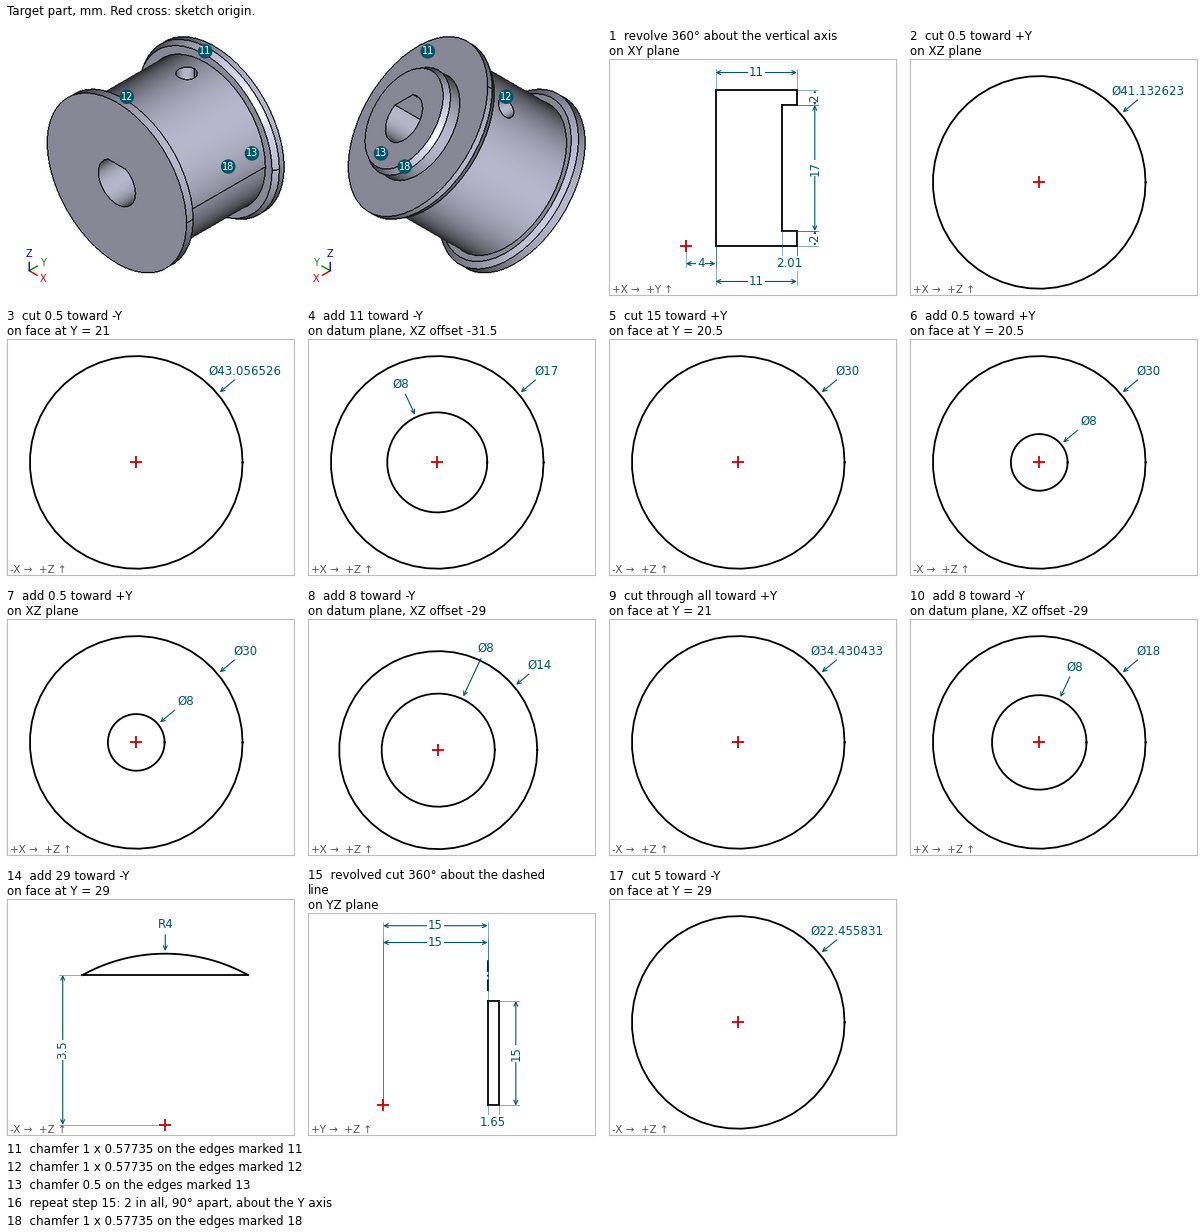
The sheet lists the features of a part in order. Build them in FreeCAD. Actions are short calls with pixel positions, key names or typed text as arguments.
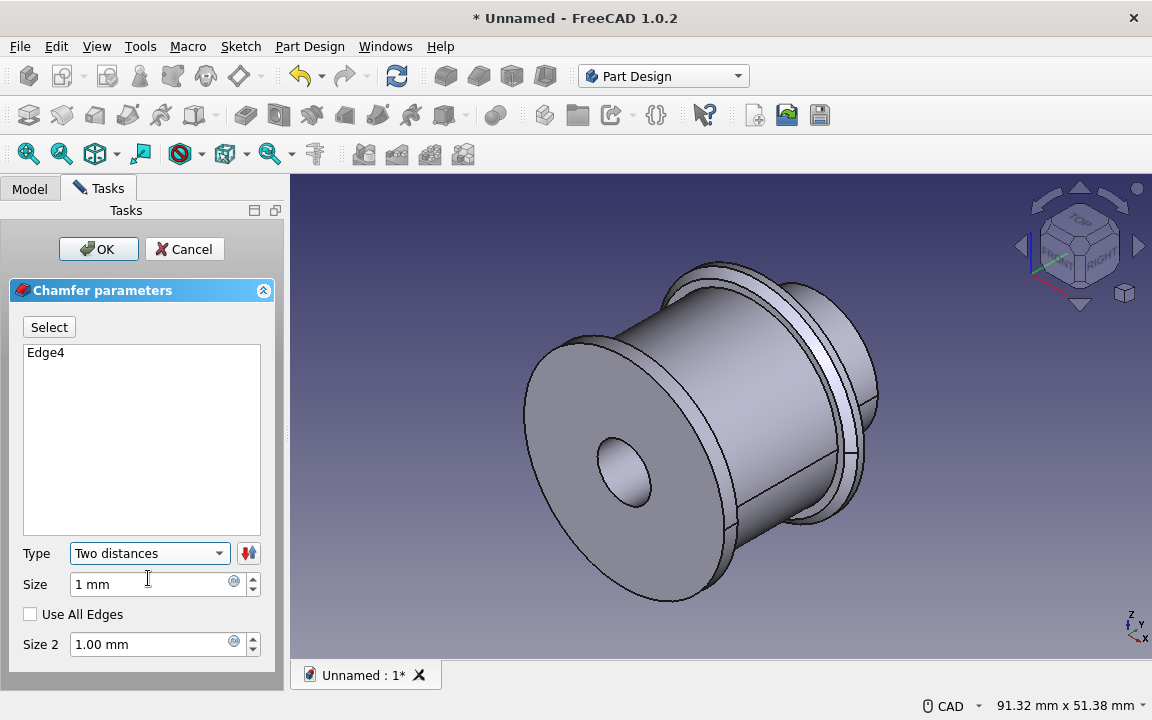
triple_click(158, 644)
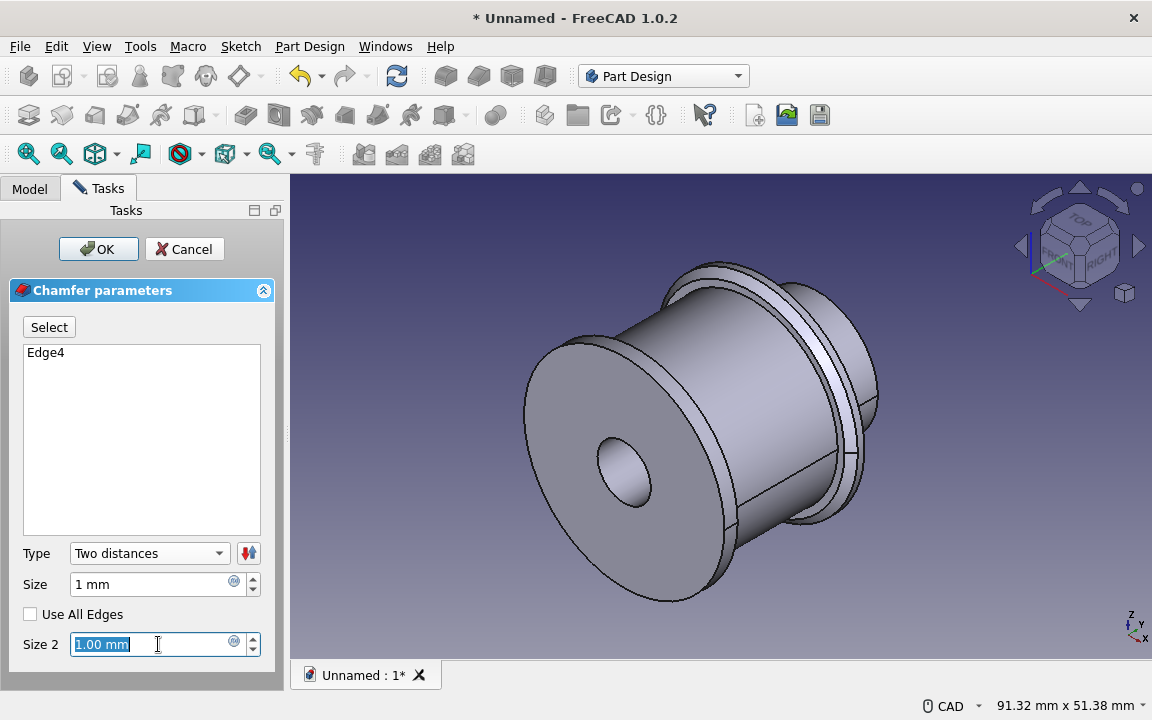
text(0.57735)
key(Tab)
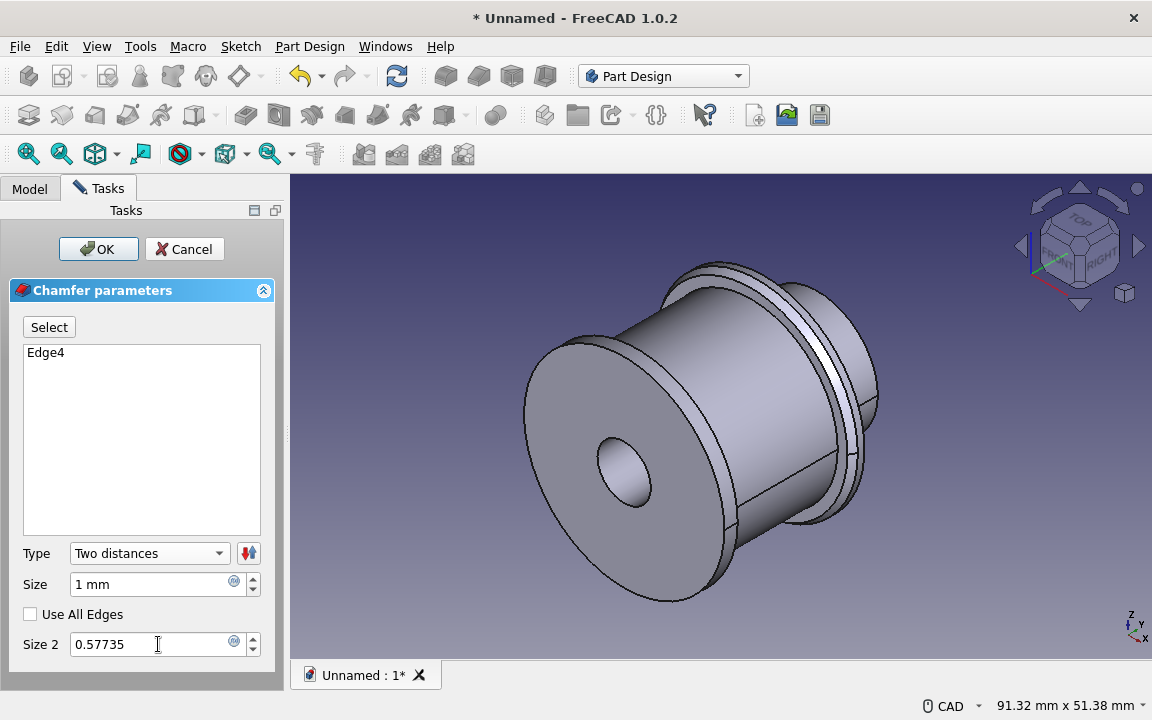
click(99, 249)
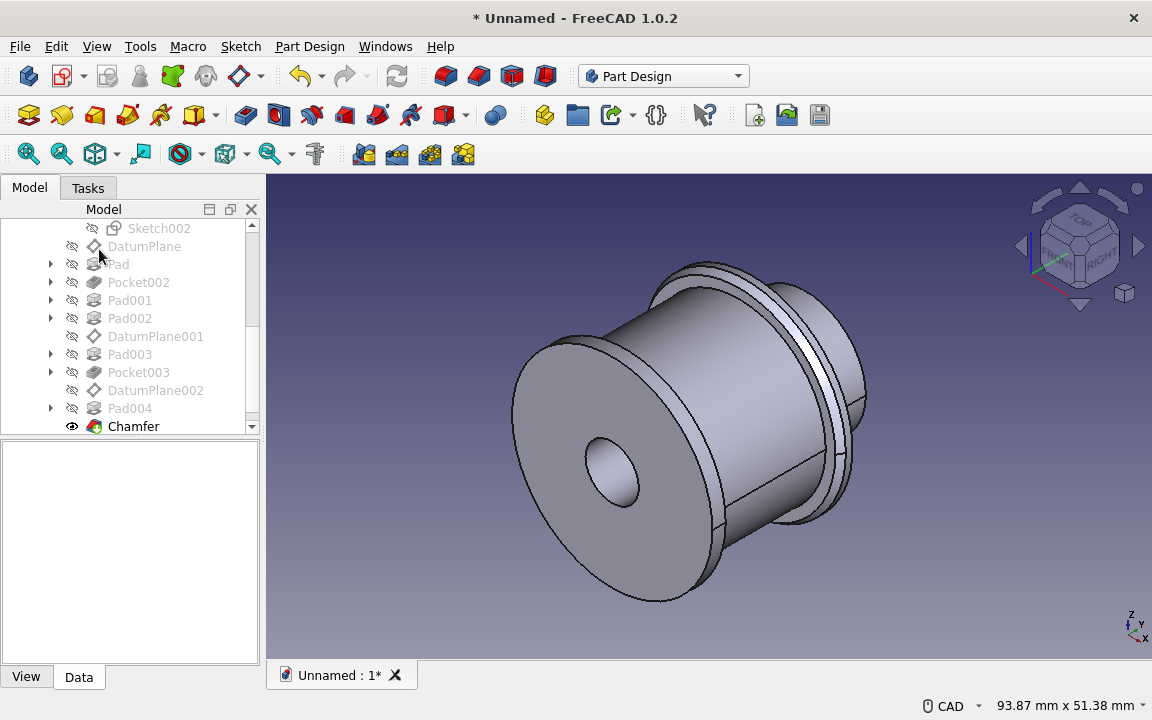
key(2)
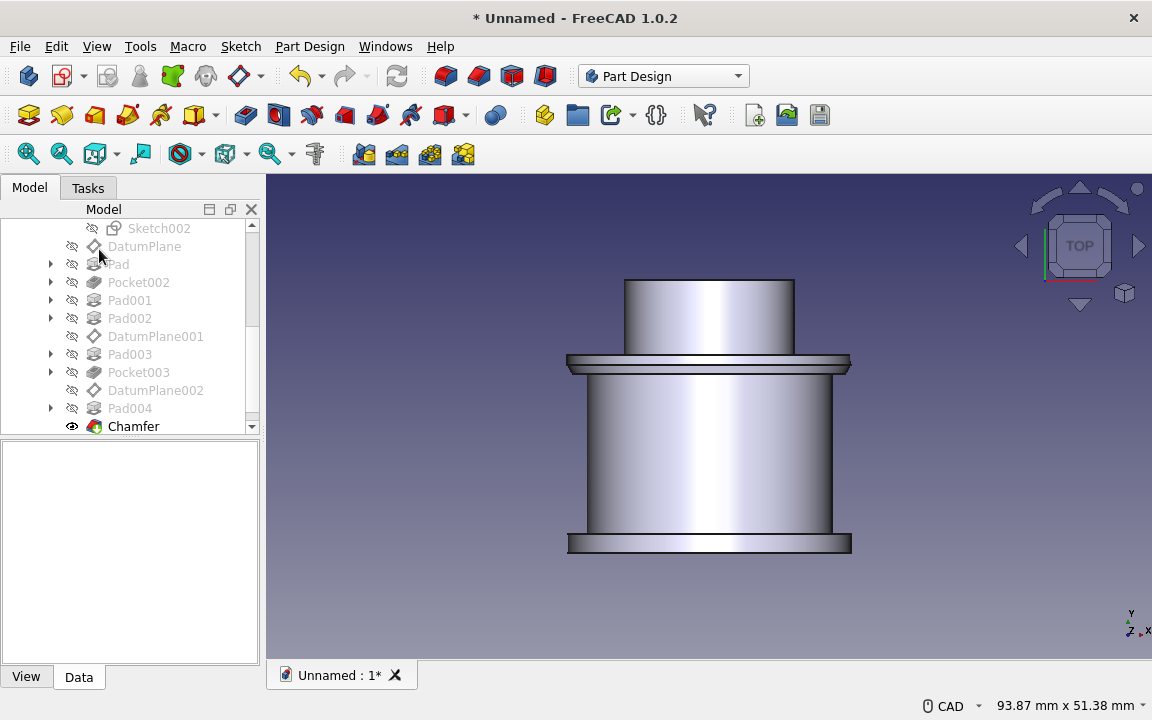
click(594, 533)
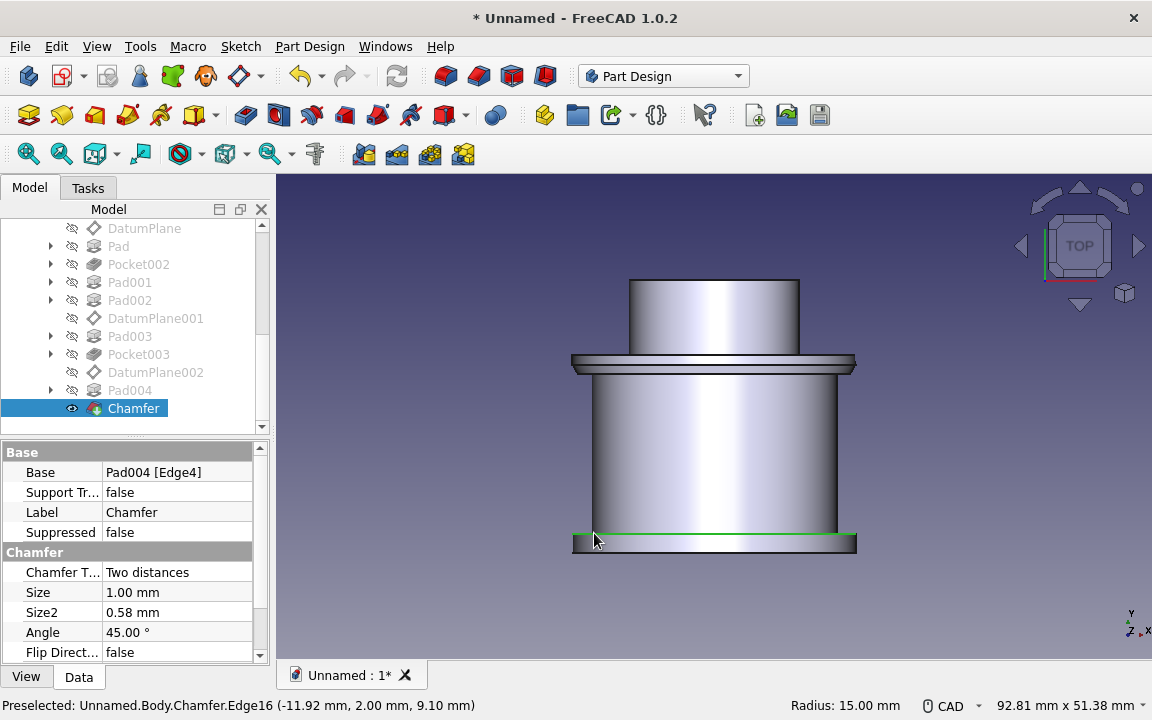
click(479, 76)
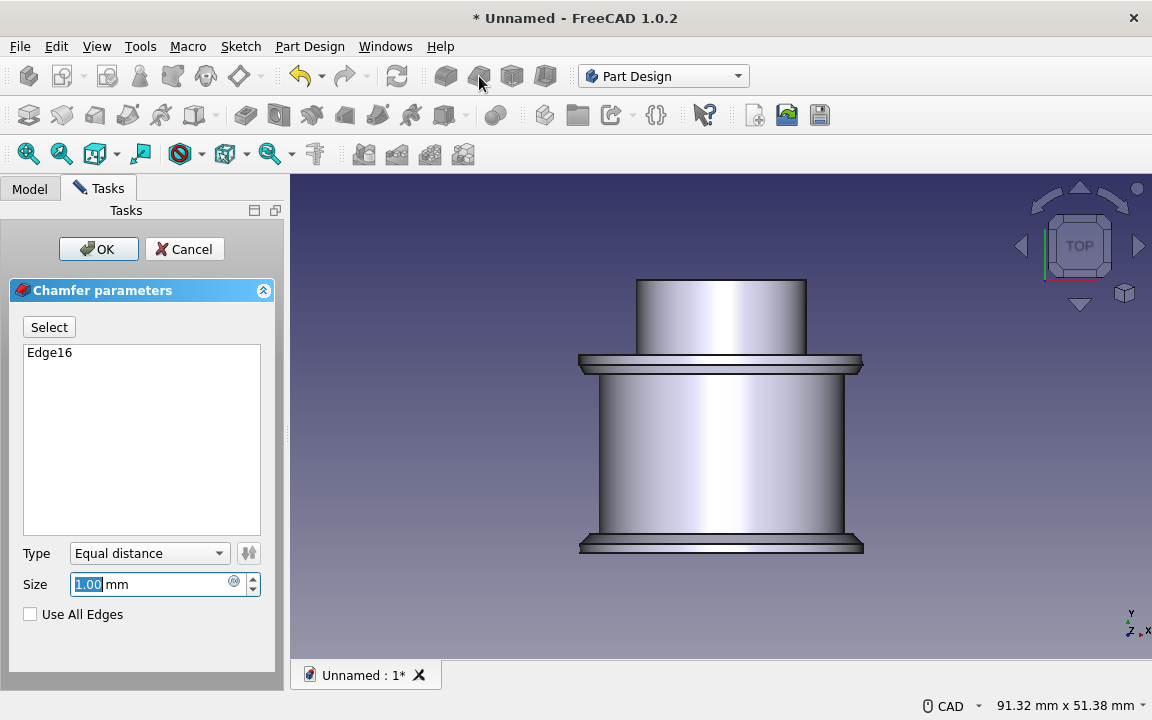
text(1)
key(Tab)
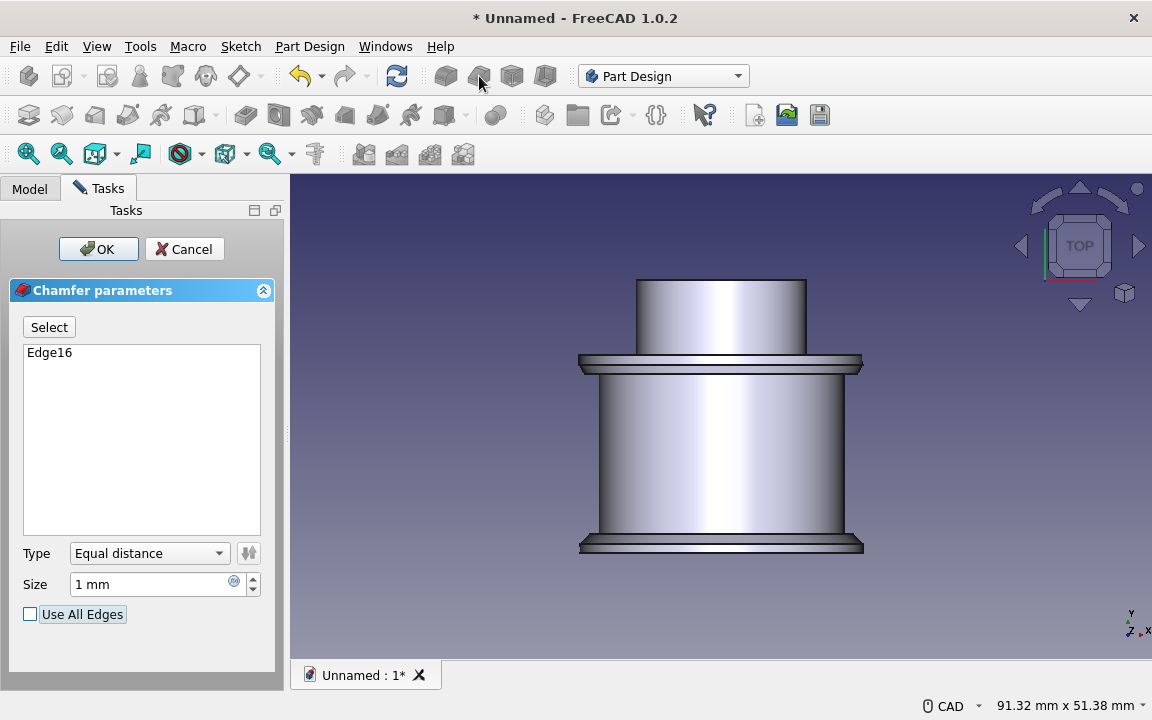
click(150, 554)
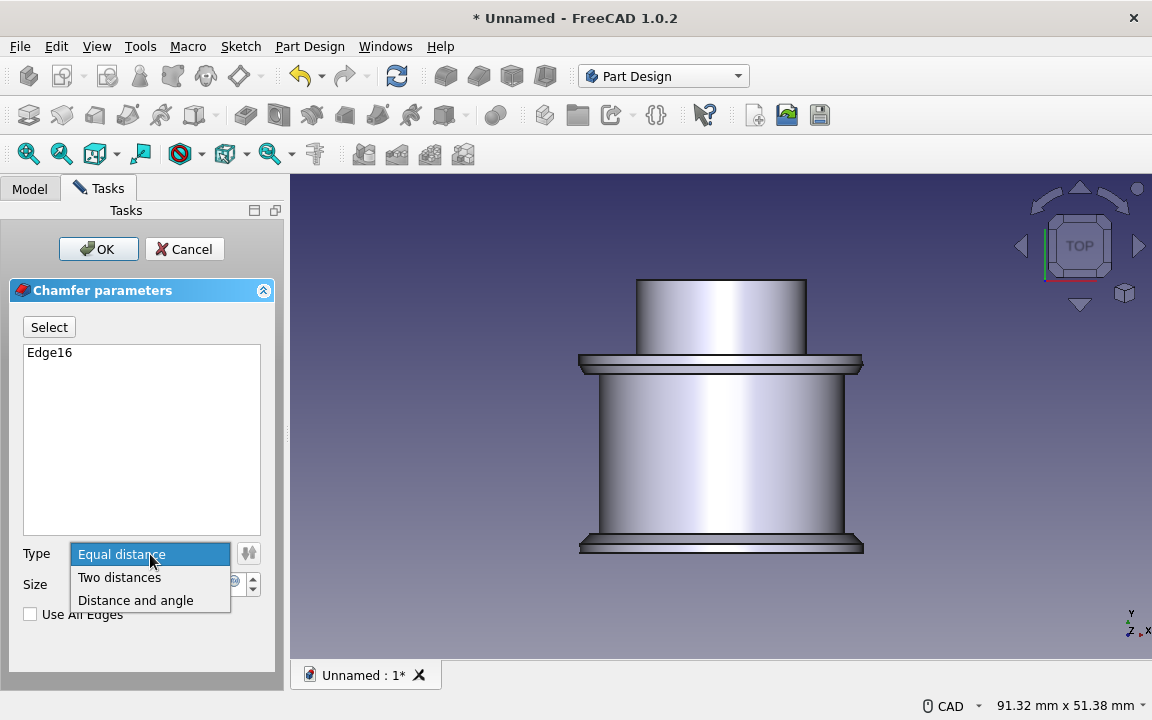
click(148, 578)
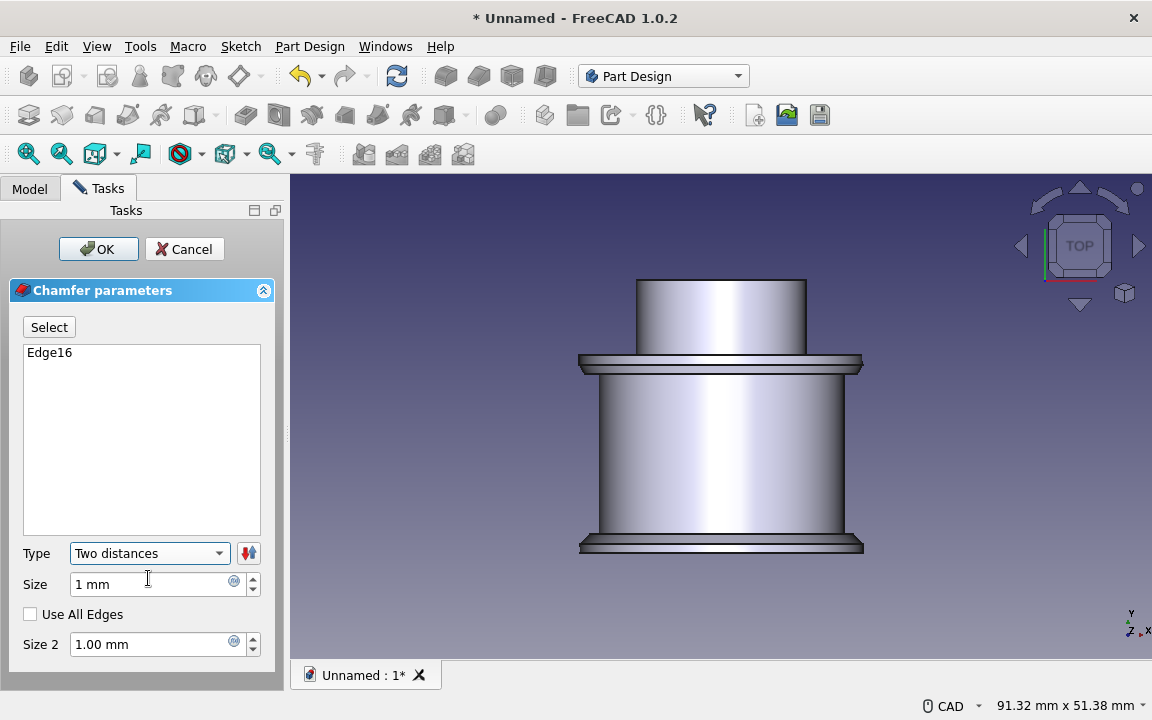
triple_click(158, 644)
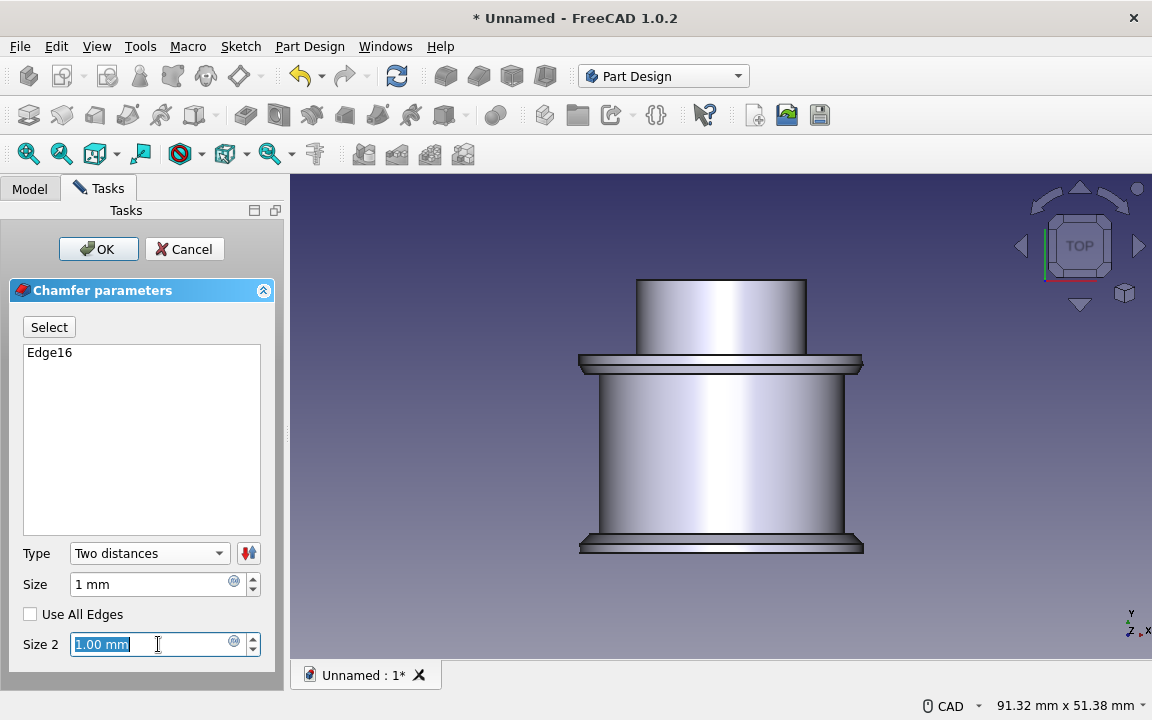
text(0.57735)
key(Tab)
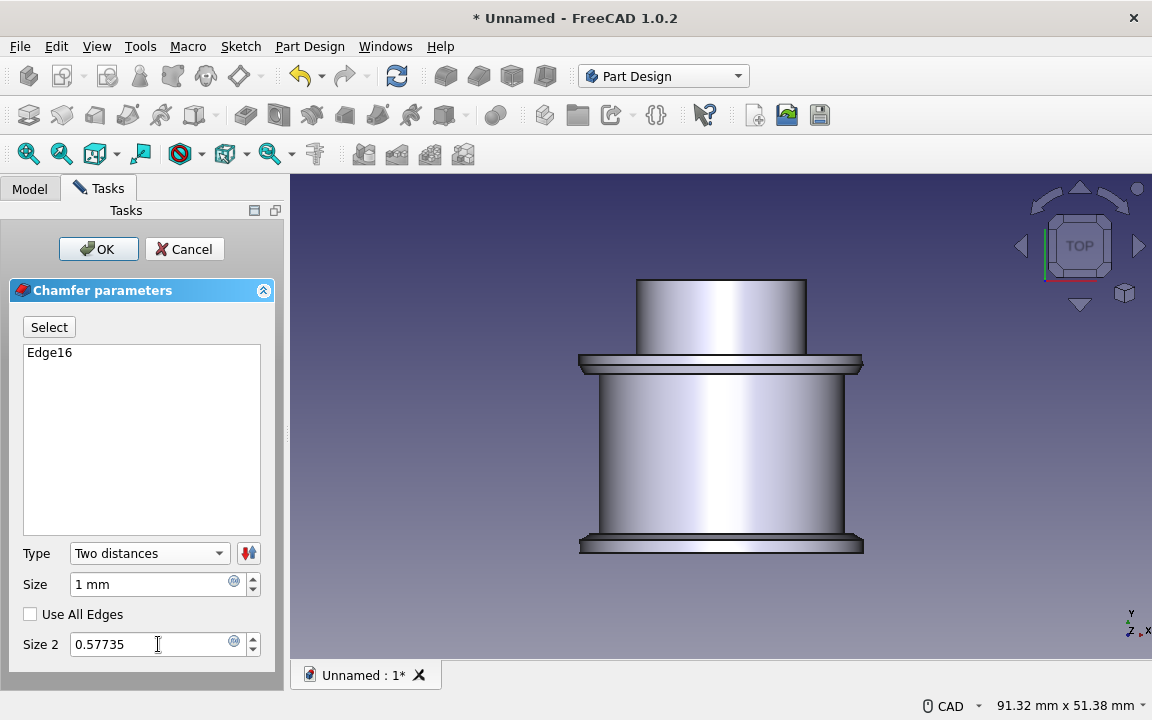
click(99, 249)